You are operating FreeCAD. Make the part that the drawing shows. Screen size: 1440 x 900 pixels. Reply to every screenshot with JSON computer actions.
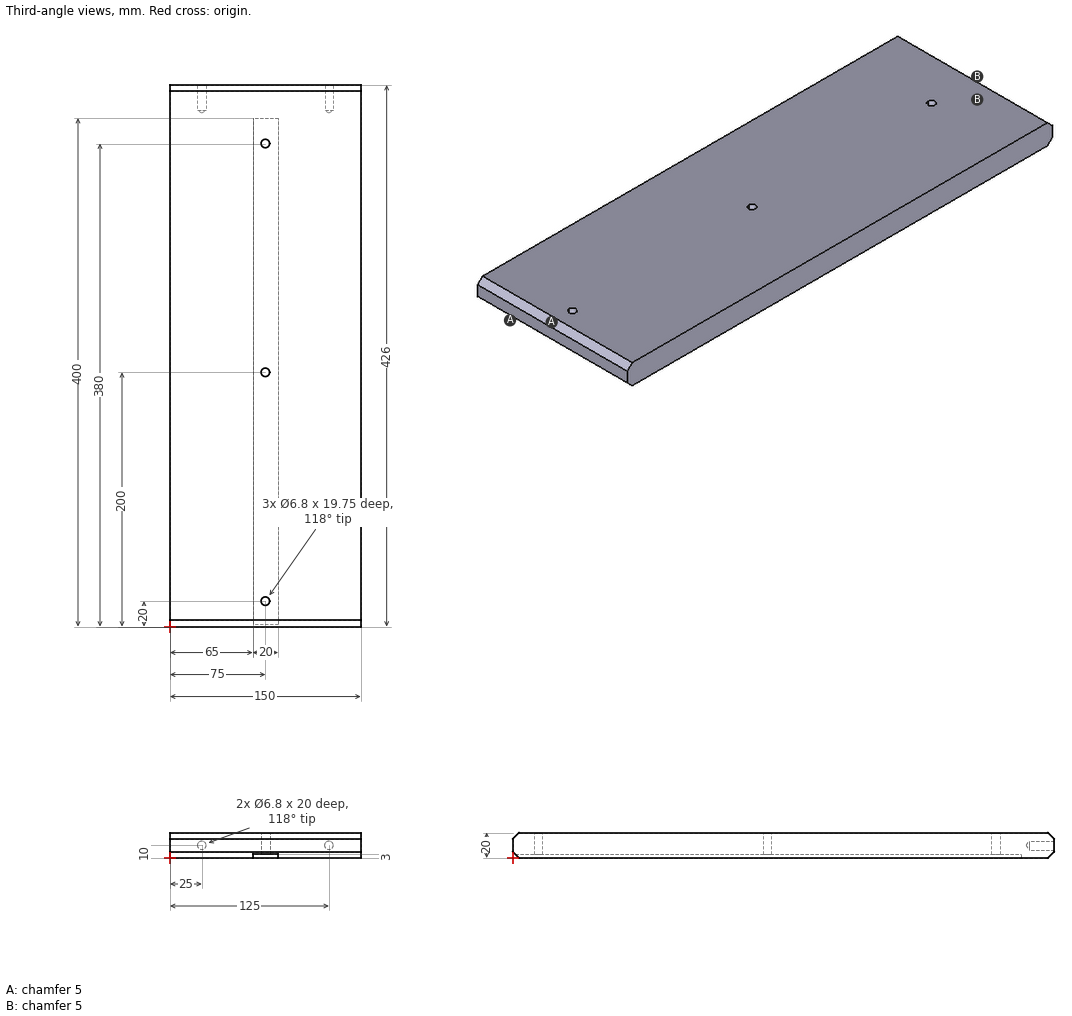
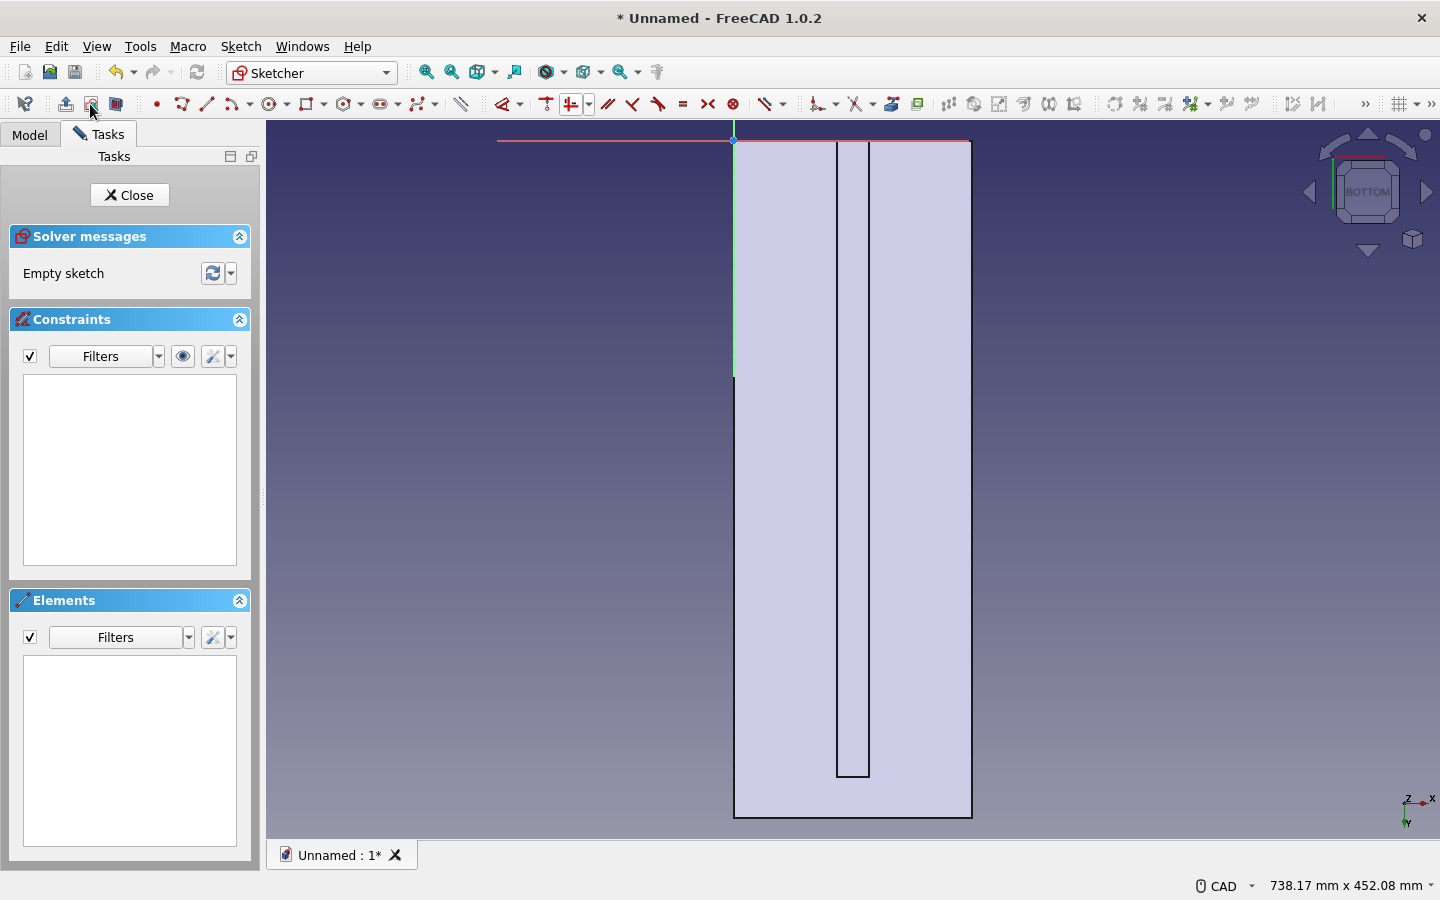
{"action": "scroll", "coordinate": [732, 633], "scroll_direction": "down", "scroll_amount": 1}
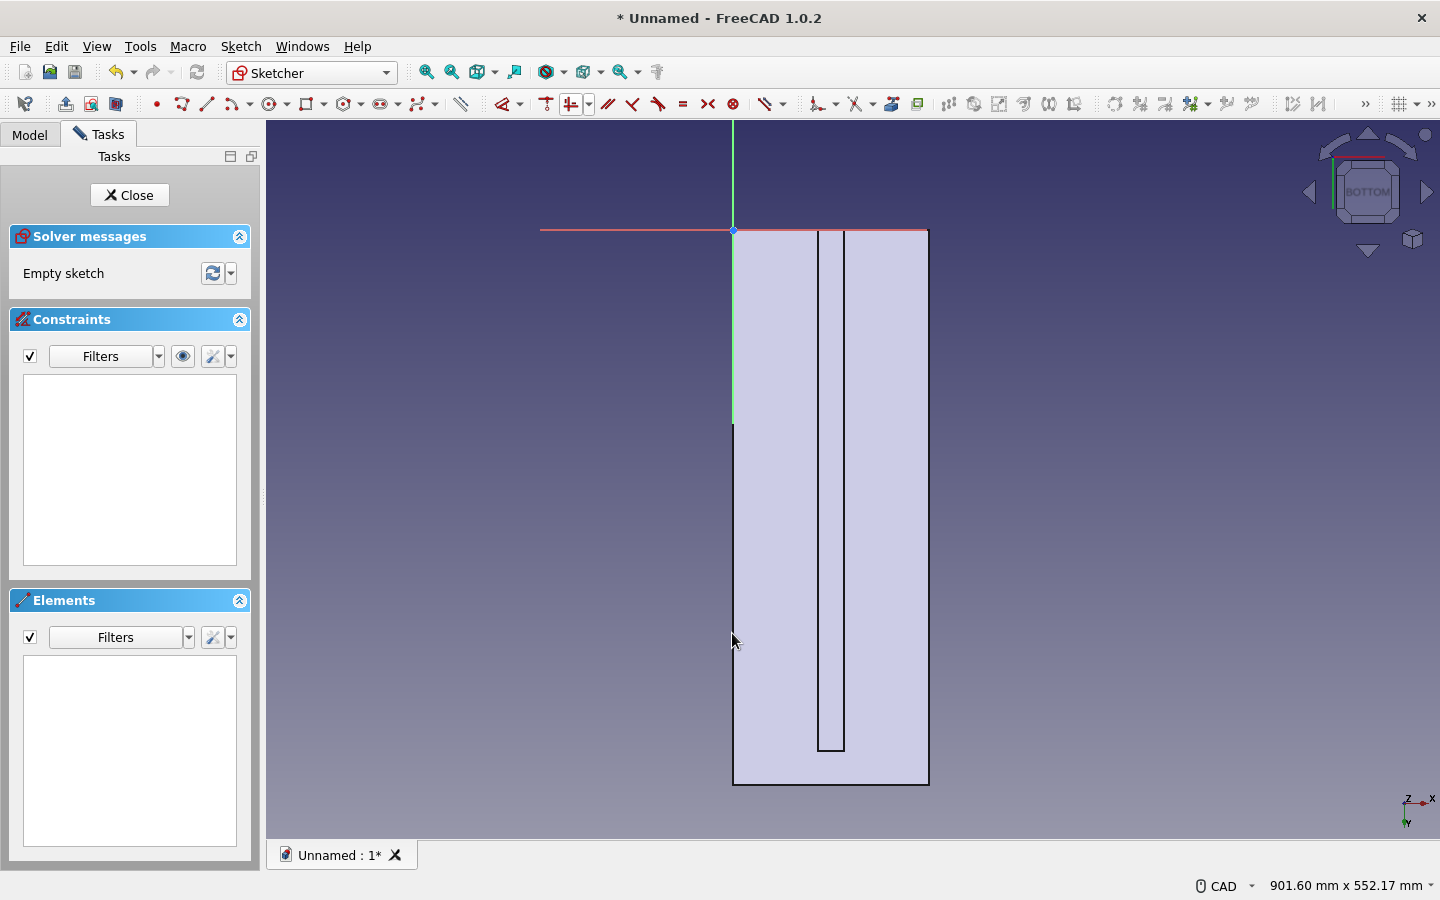
{"action": "left_click", "coordinate": [268, 104]}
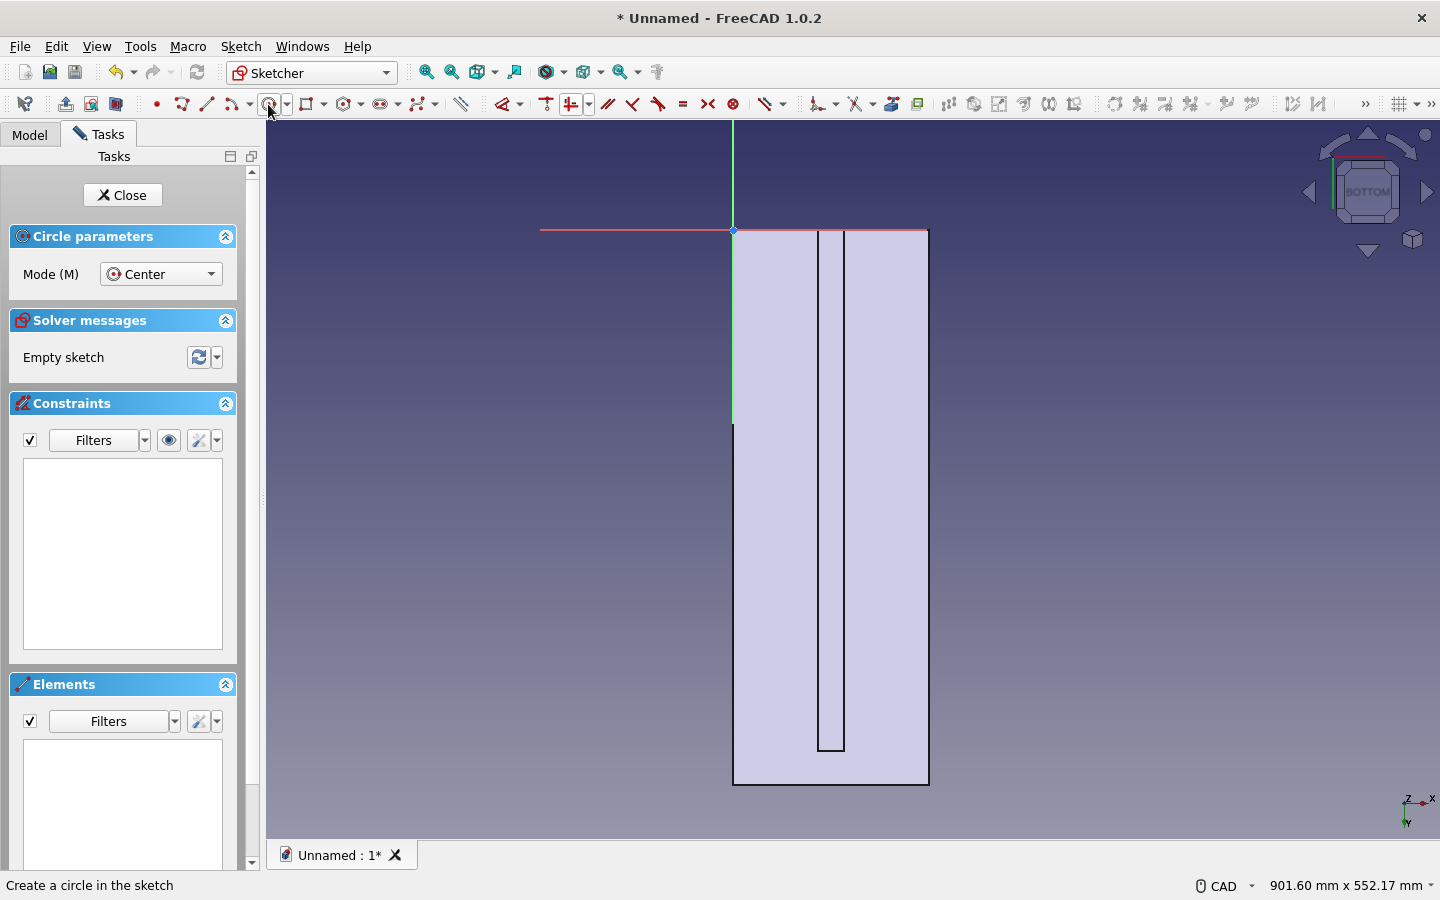
{"action": "scroll", "coordinate": [831, 256], "scroll_direction": "up", "scroll_amount": 9}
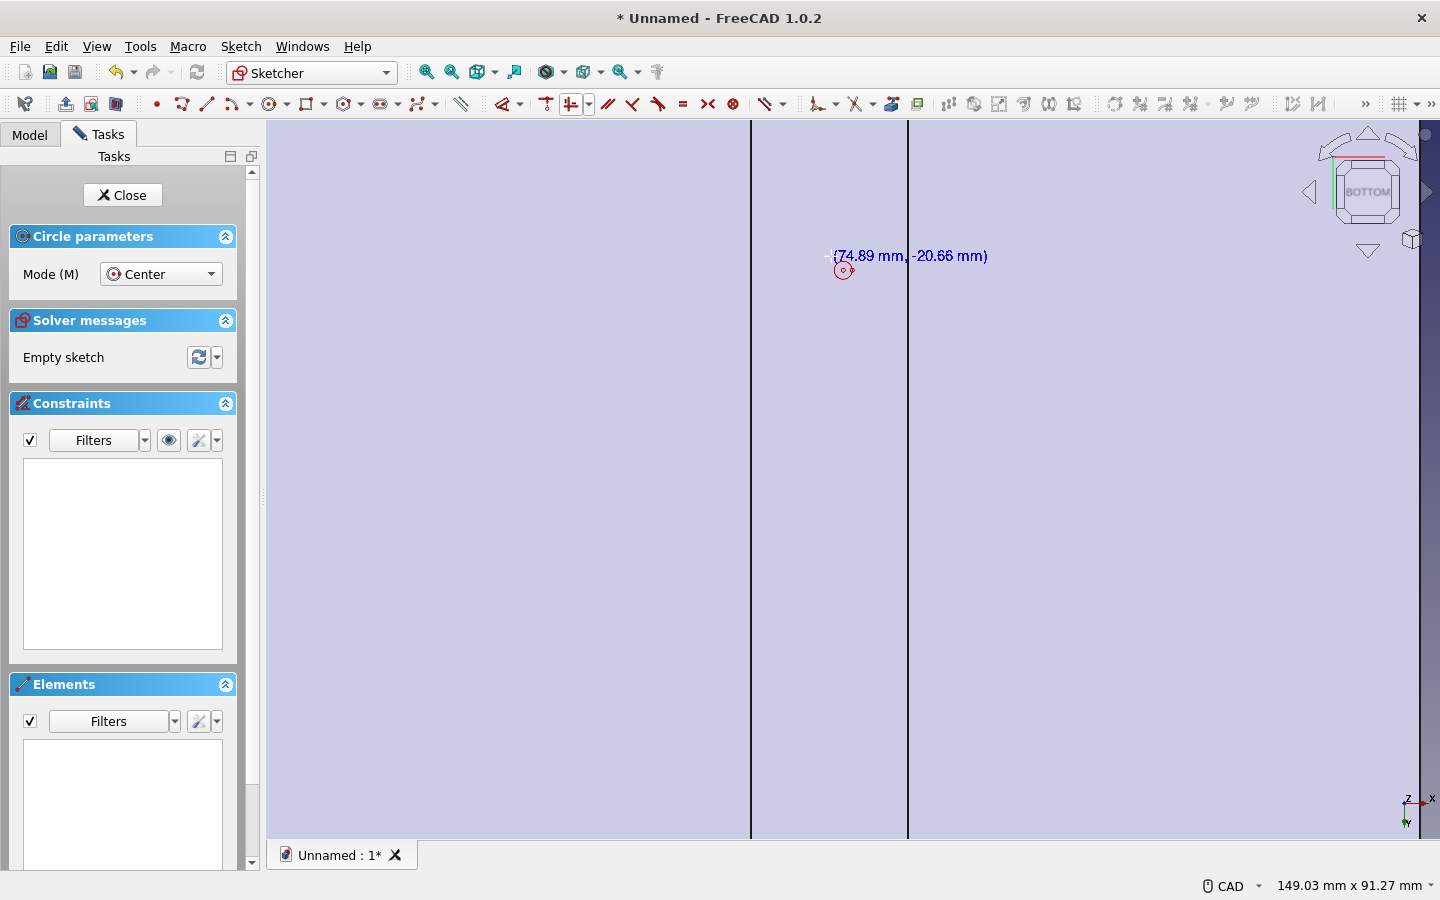
{"action": "scroll", "coordinate": [831, 256], "scroll_direction": "down", "scroll_amount": 9}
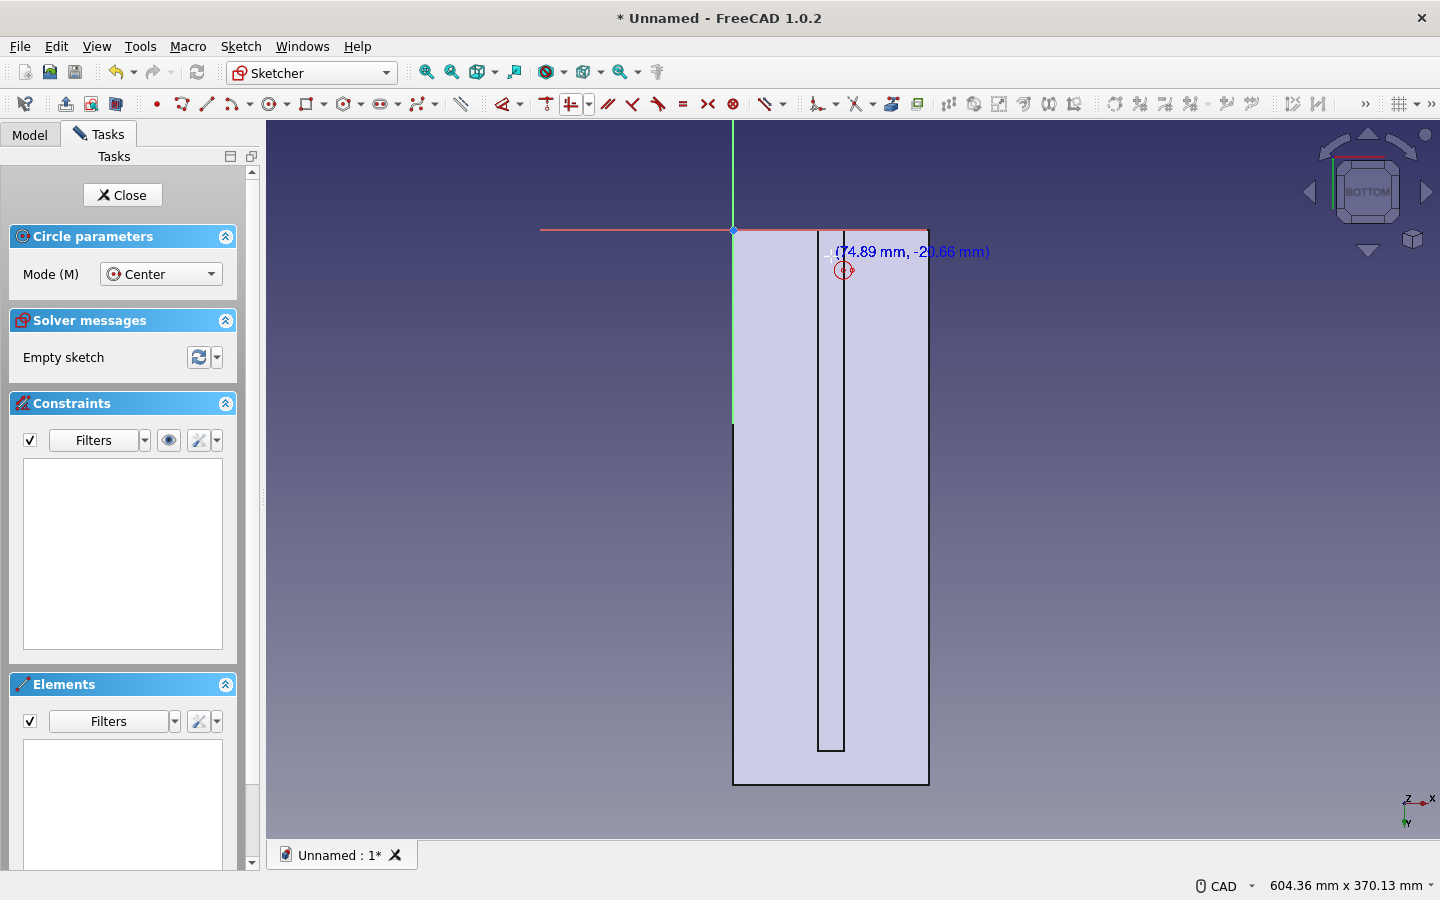
{"action": "left_click", "coordinate": [831, 256]}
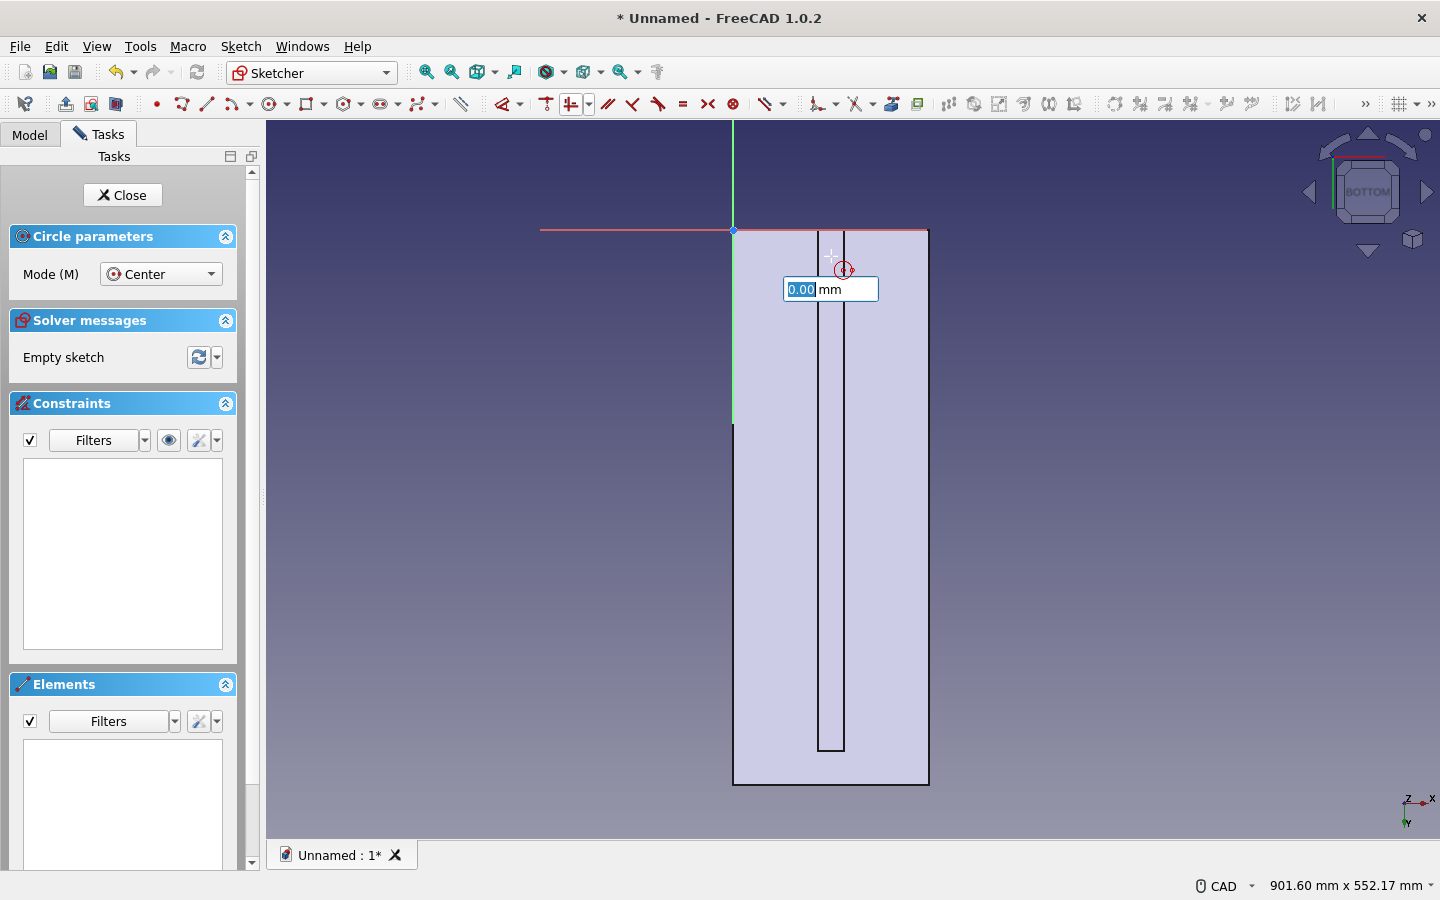
{"action": "scroll", "coordinate": [834, 253], "scroll_direction": "up", "scroll_amount": 7}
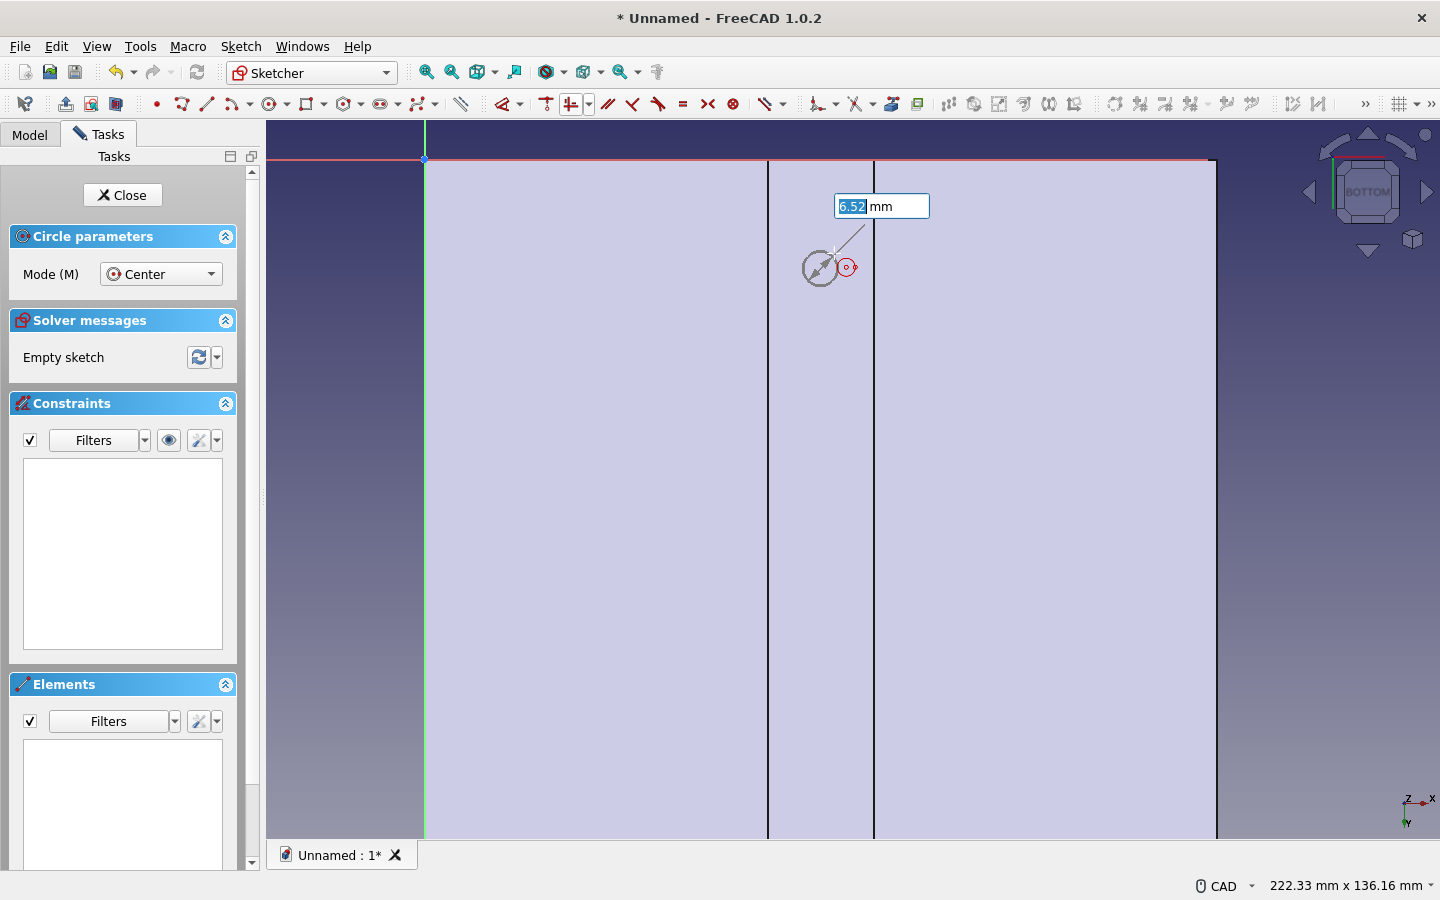
{"action": "left_click", "coordinate": [834, 252]}